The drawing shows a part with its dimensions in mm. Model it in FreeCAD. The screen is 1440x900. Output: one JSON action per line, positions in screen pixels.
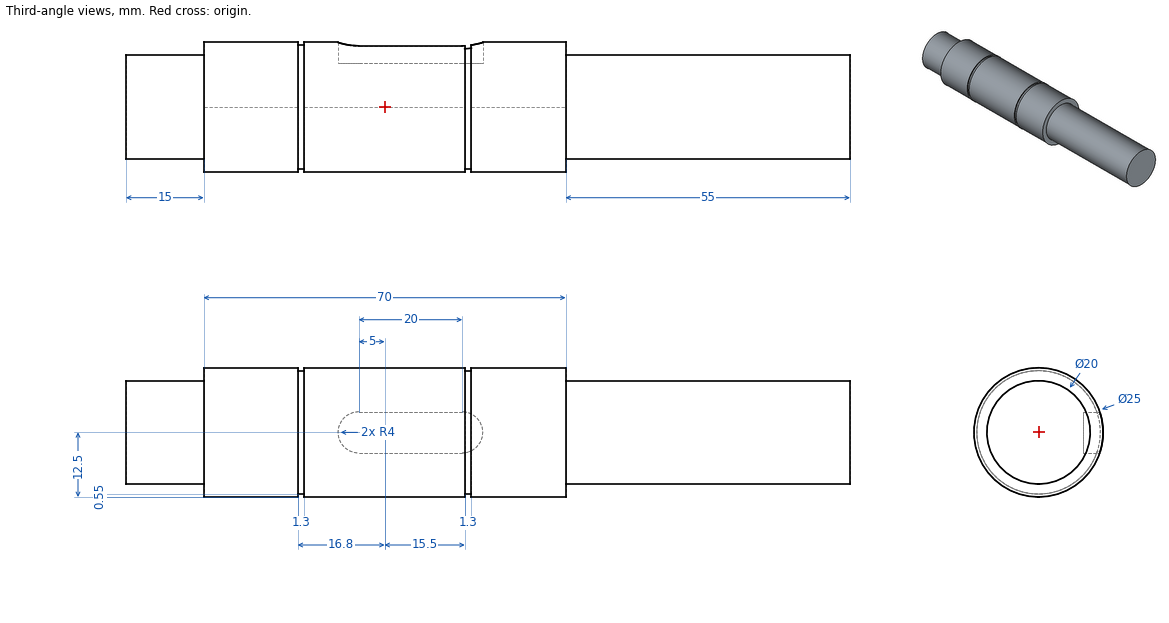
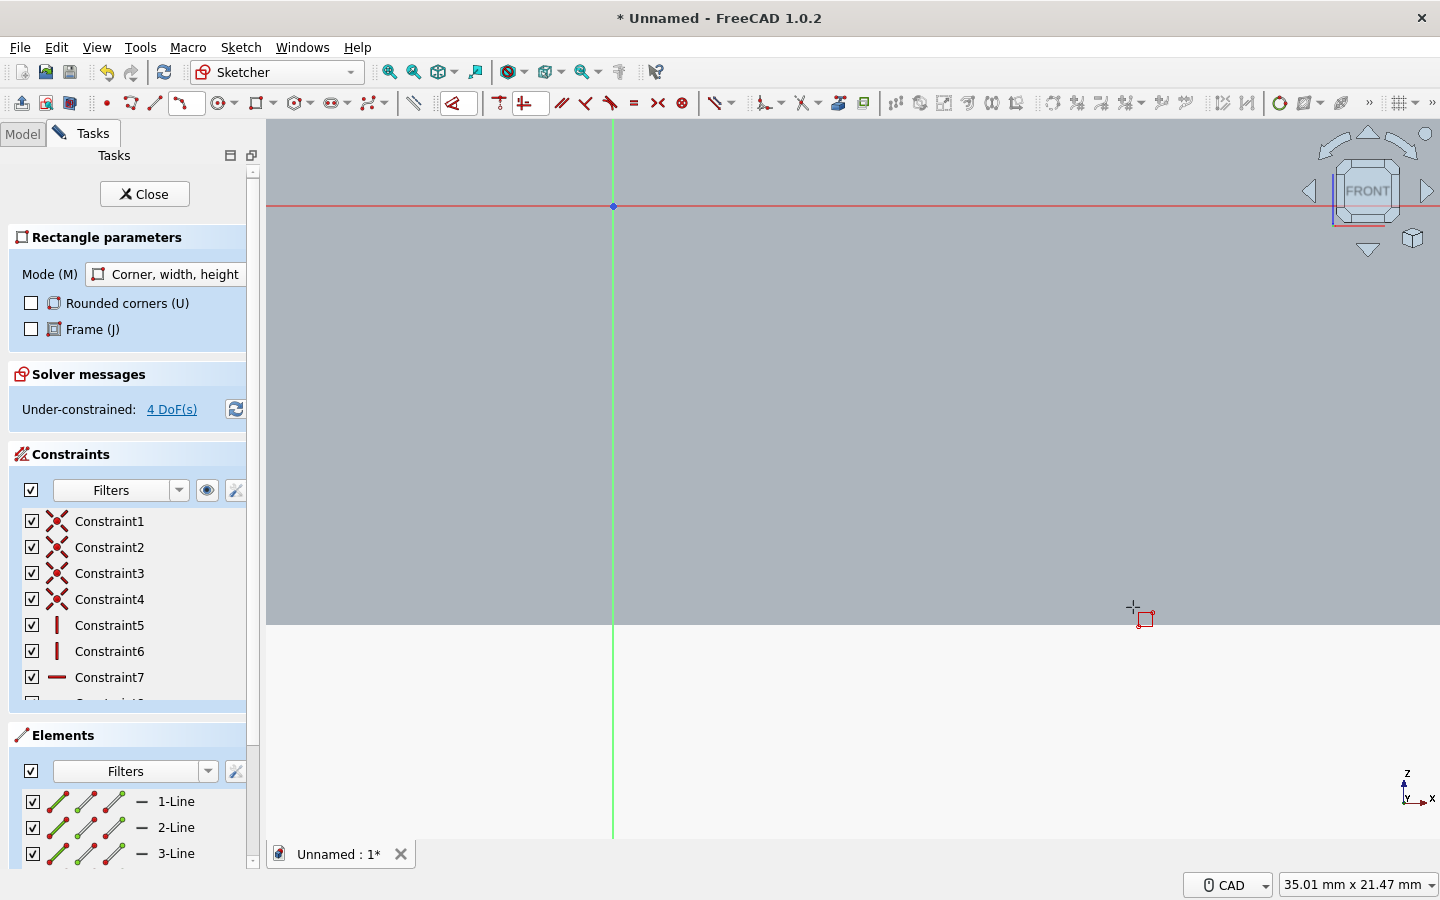
{"action": "left_click", "coordinate": [1133, 607]}
{"action": "left_click", "coordinate": [1176, 626]}
{"action": "key", "text": "Escape"}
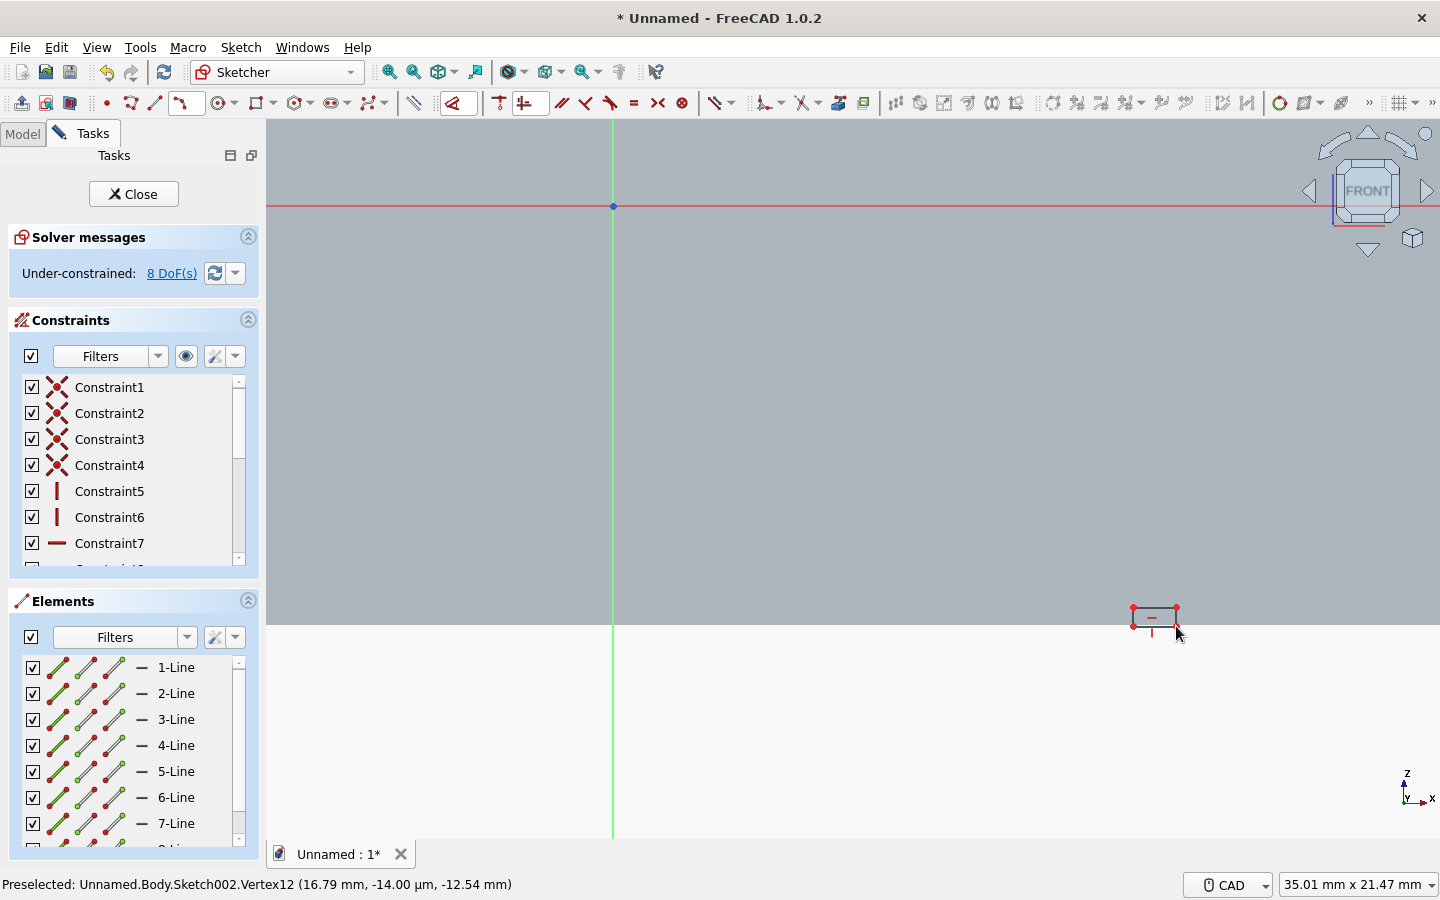
{"action": "scroll", "coordinate": [1133, 607], "scroll_direction": "down", "scroll_amount": 2}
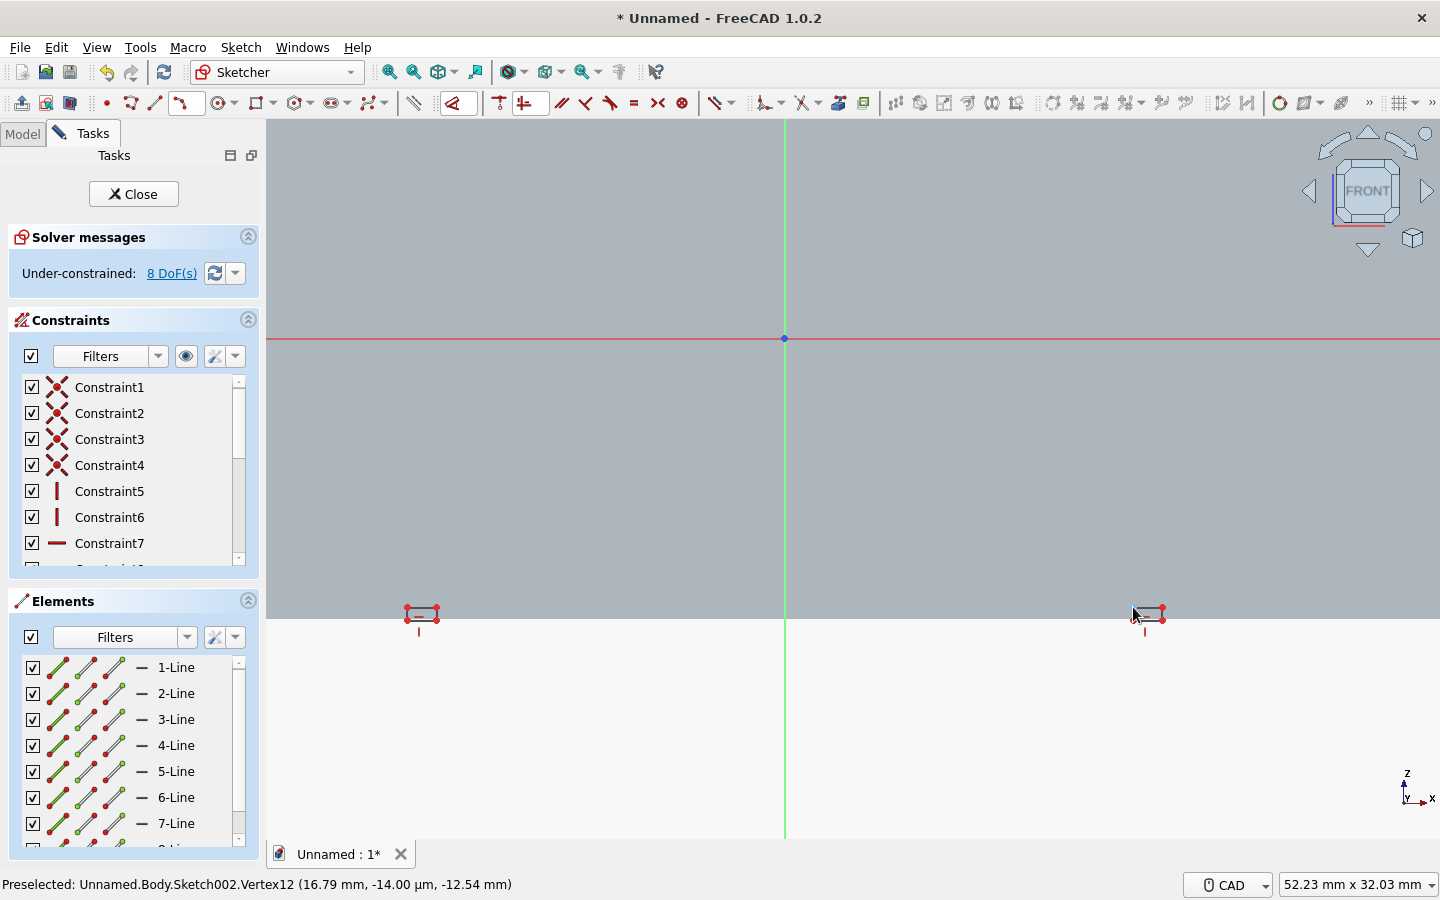
{"action": "scroll", "coordinate": [416, 621], "scroll_direction": "up", "scroll_amount": 3}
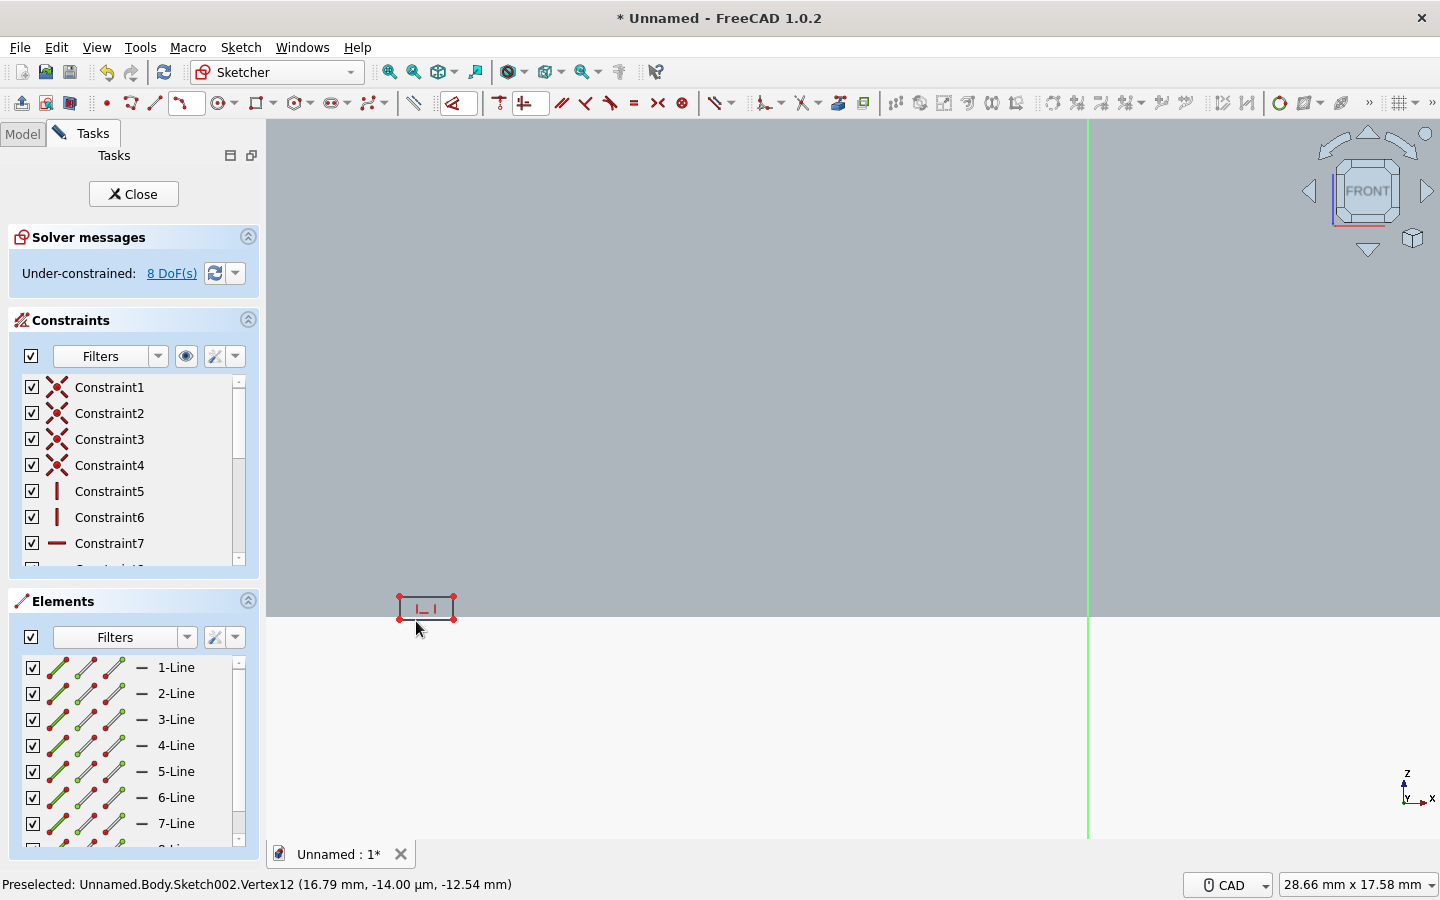
{"action": "left_click", "coordinate": [416, 620]}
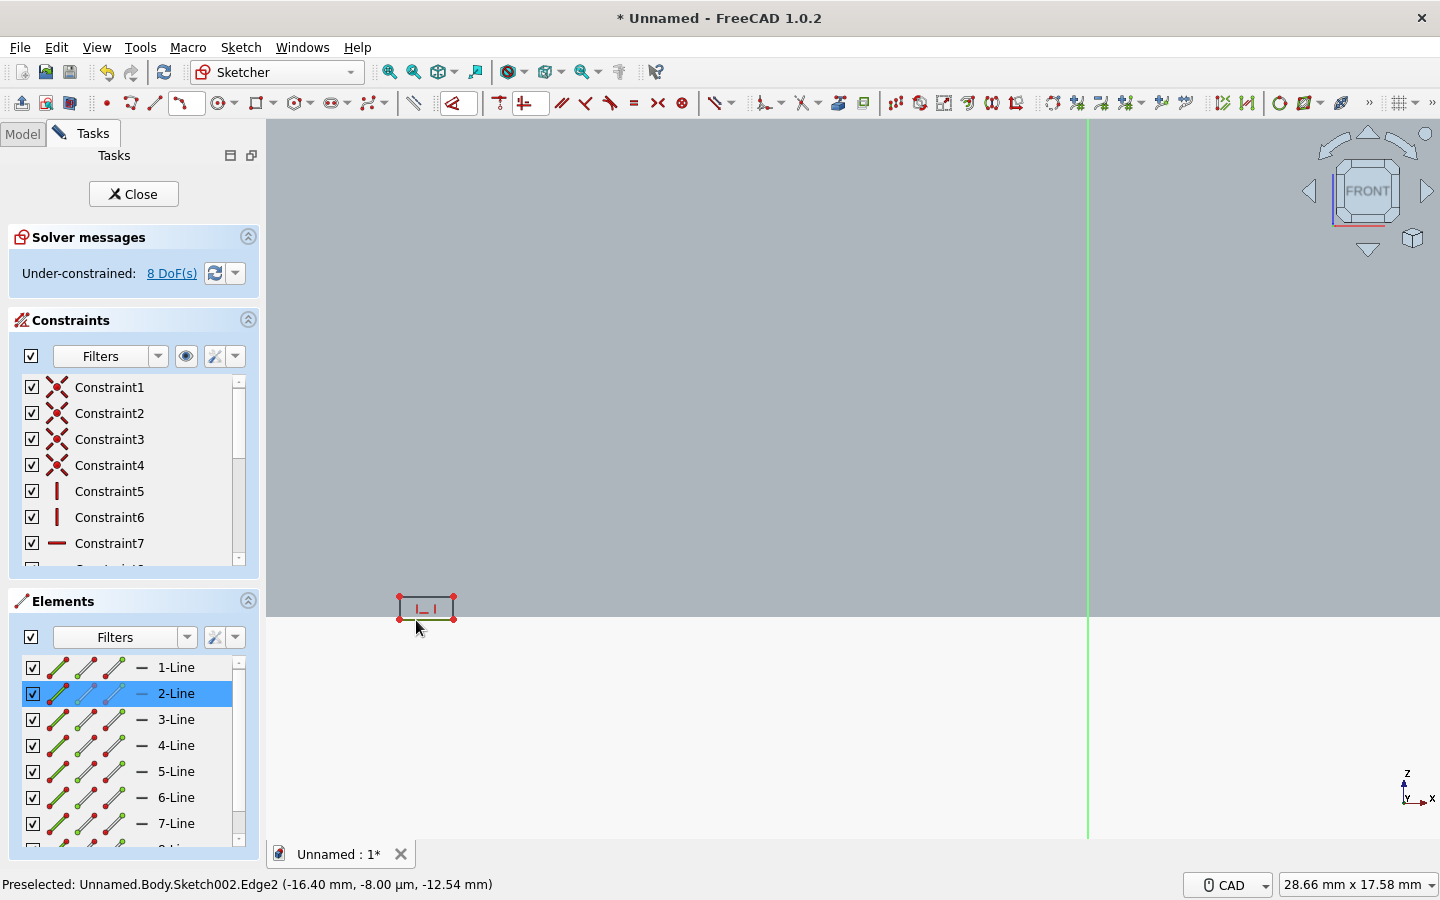
{"action": "left_click", "coordinate": [472, 104]}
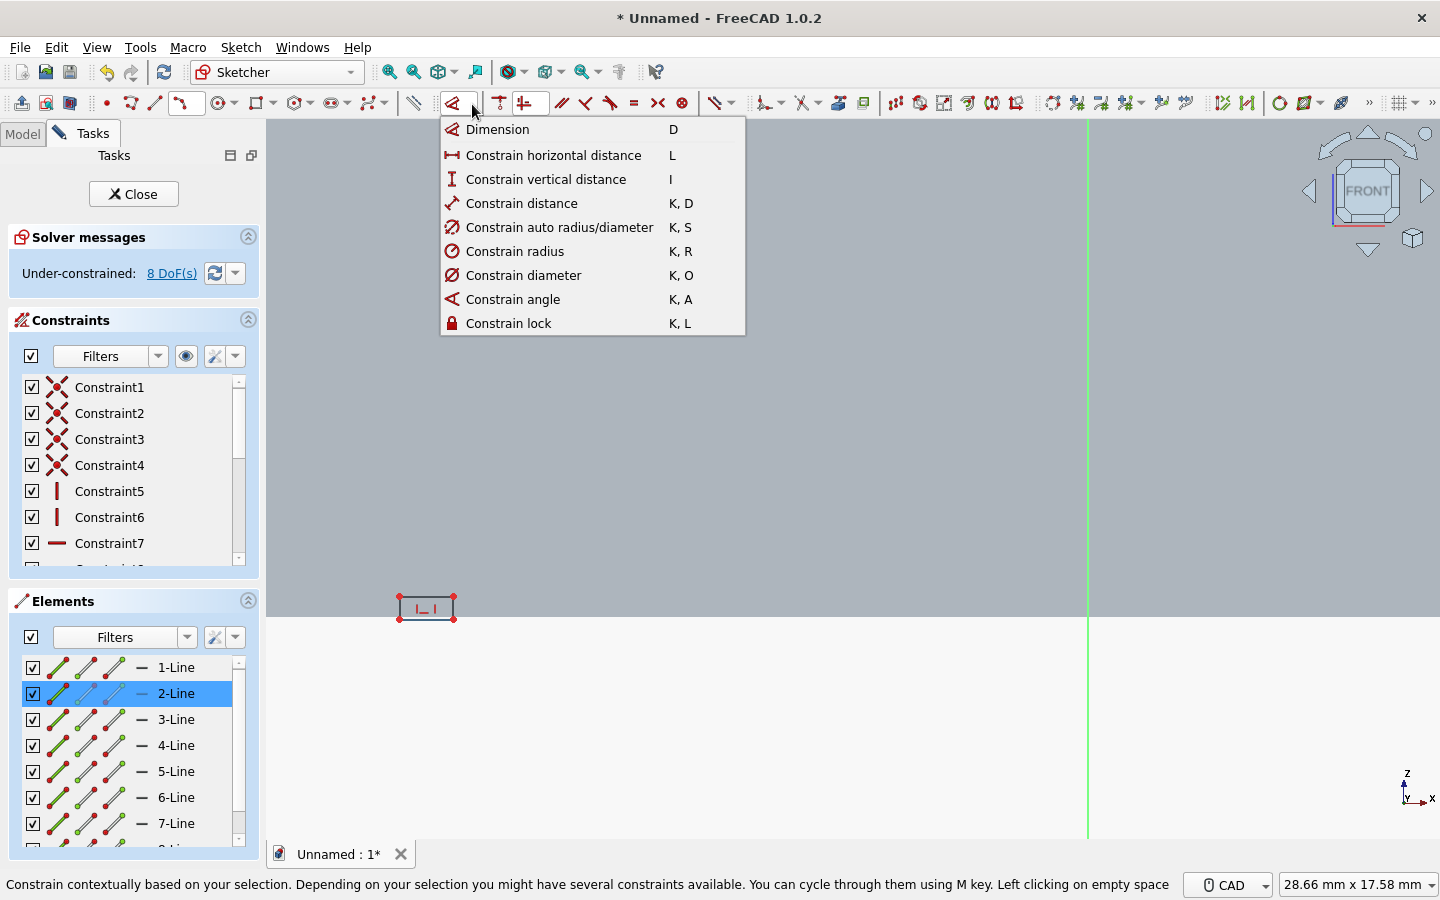
{"action": "left_click", "coordinate": [593, 155]}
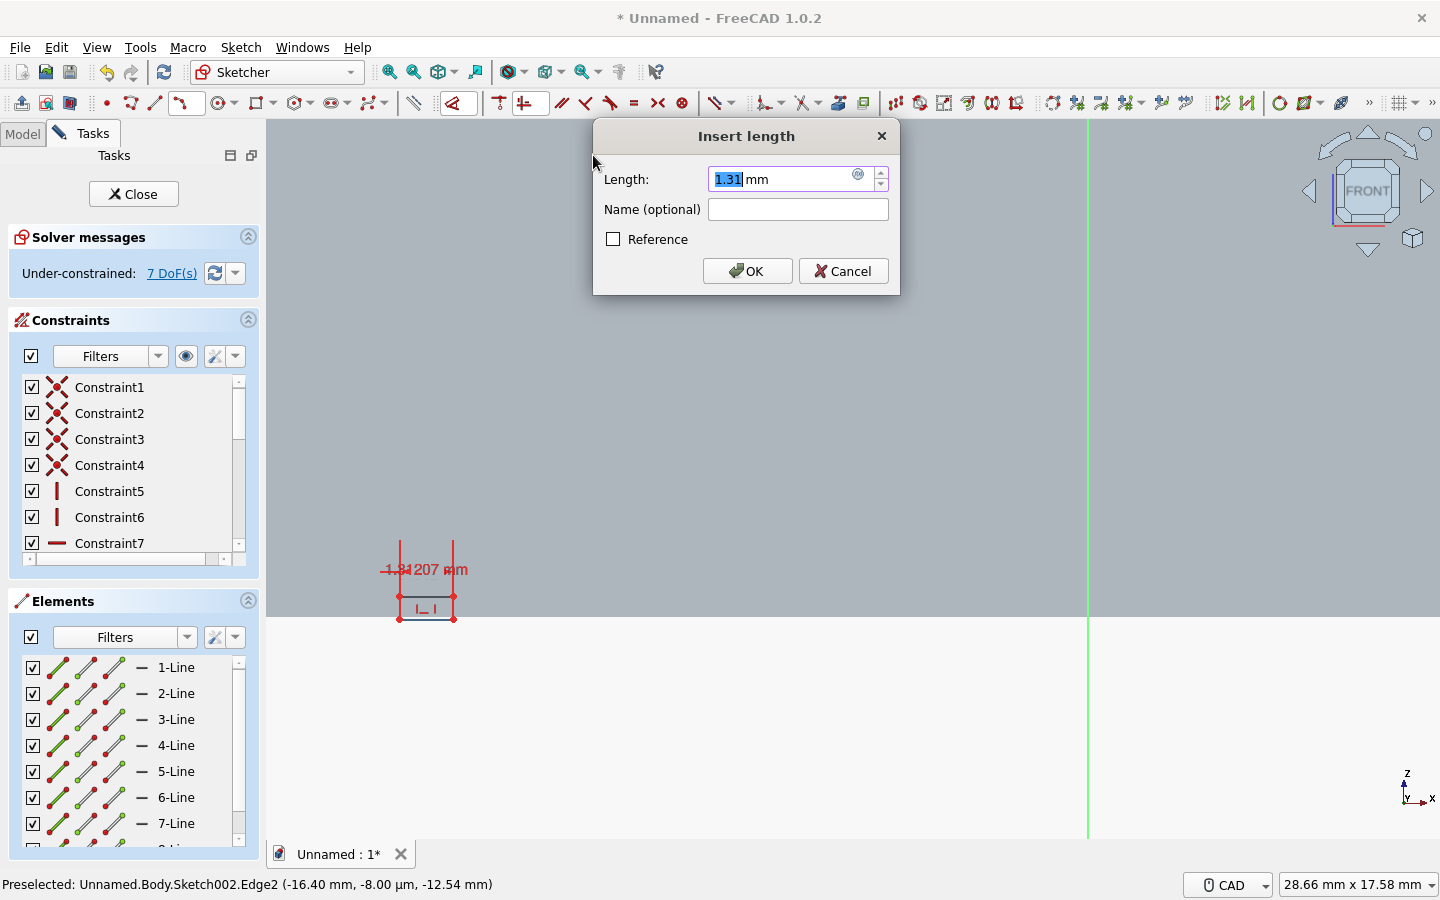
{"action": "type", "text": "1.3"}
{"action": "key", "text": "Return"}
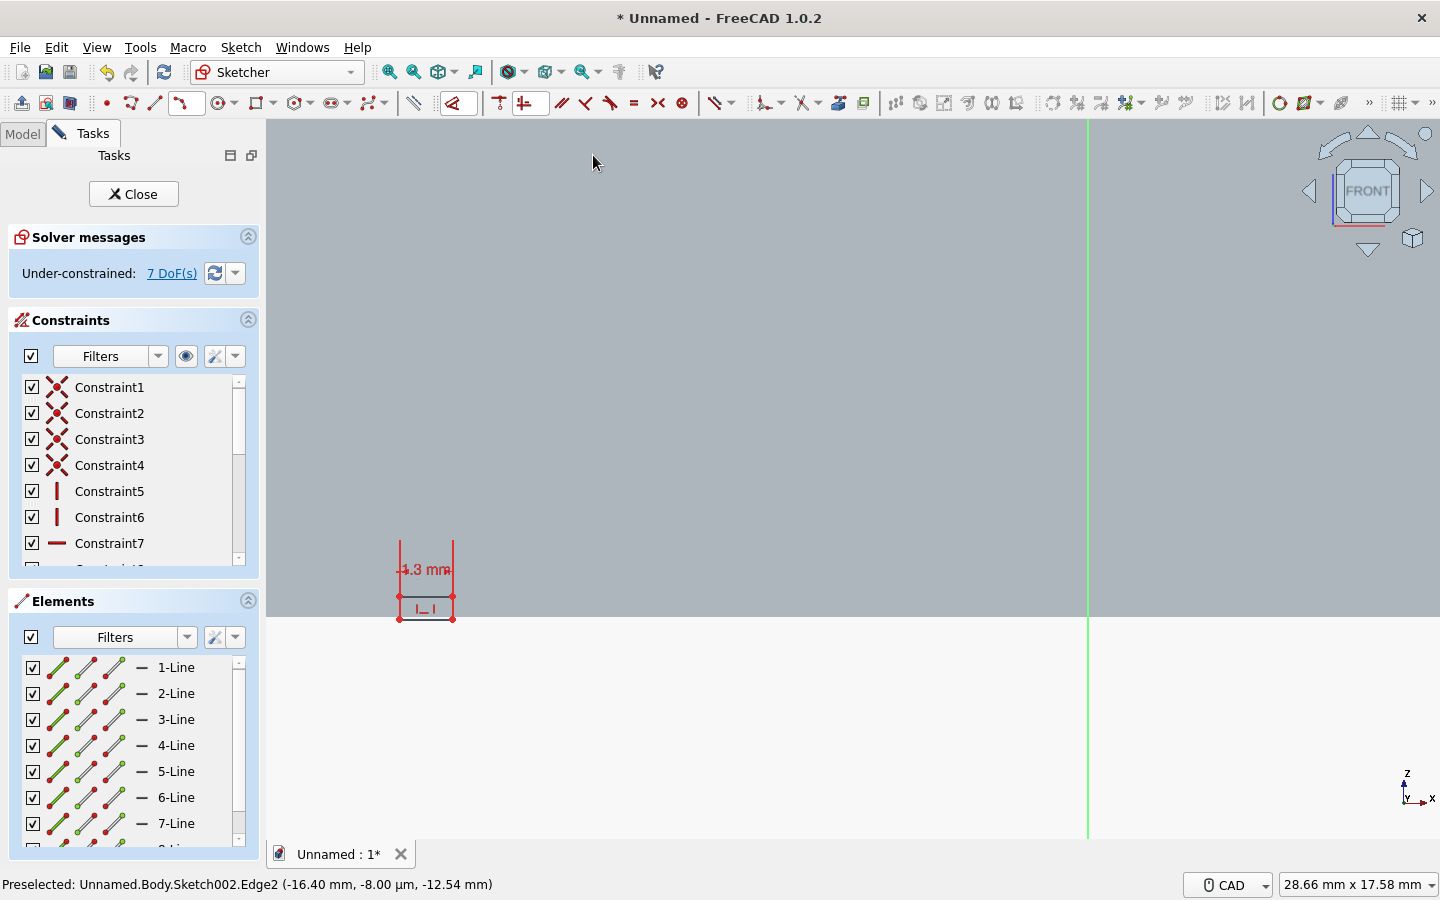
{"action": "scroll", "coordinate": [416, 621], "scroll_direction": "down", "scroll_amount": 3}